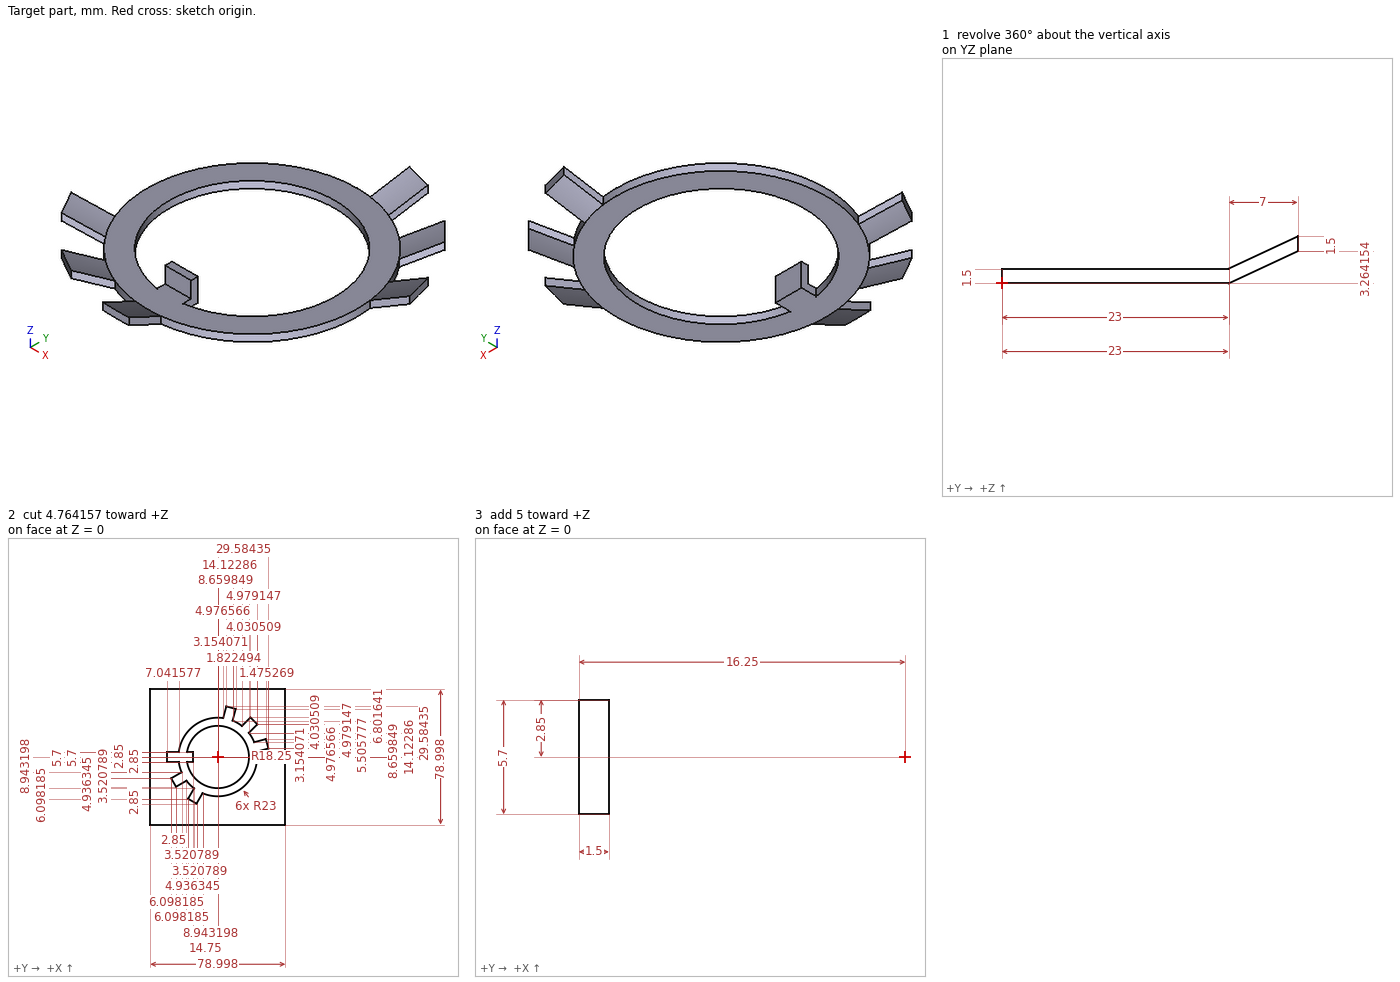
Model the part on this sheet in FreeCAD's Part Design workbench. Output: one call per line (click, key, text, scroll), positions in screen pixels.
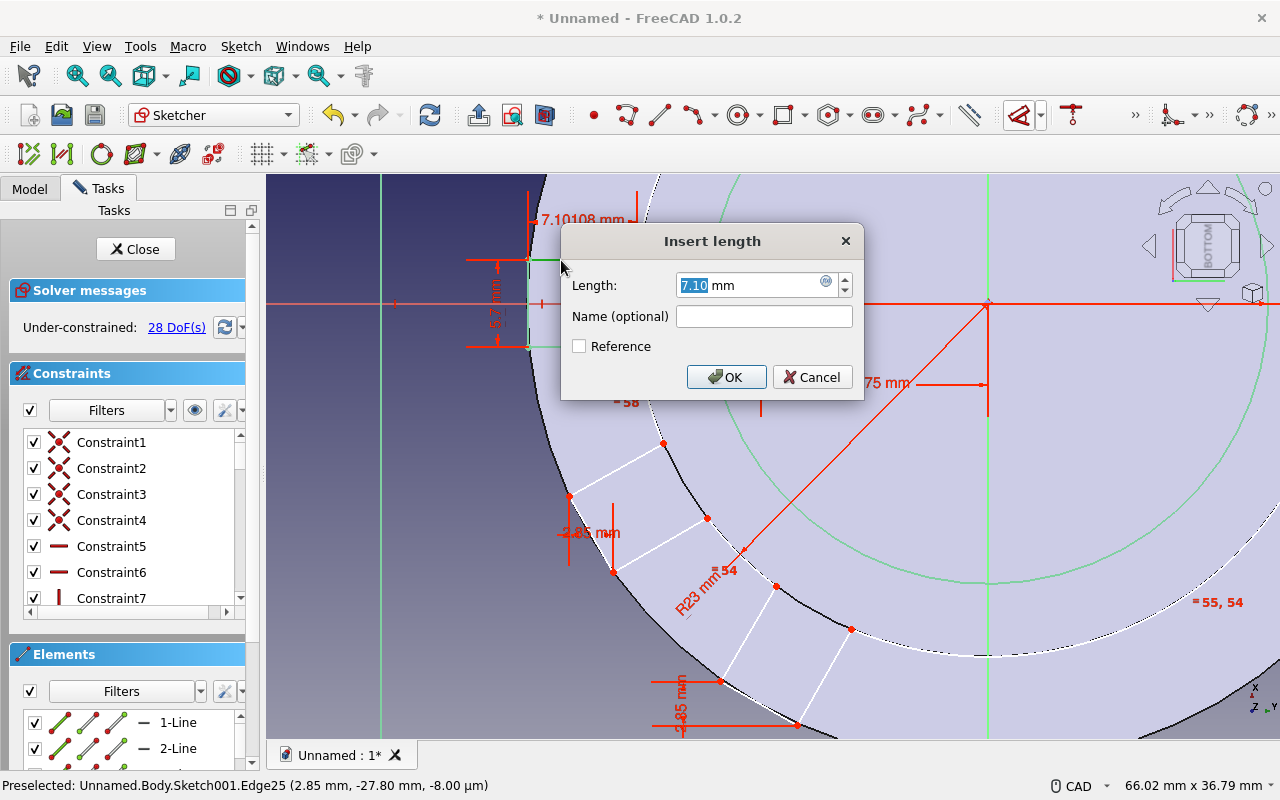
text(7.041577)
key(Return)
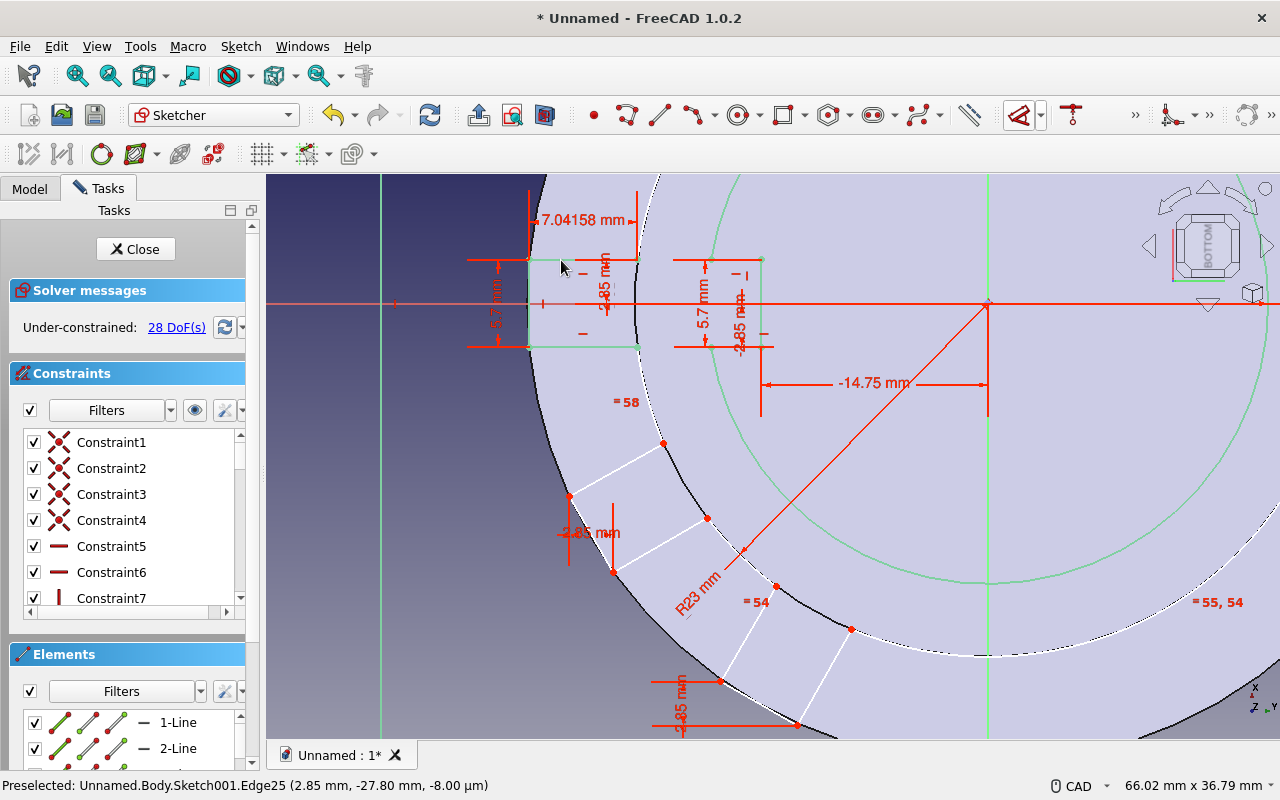
click(664, 444)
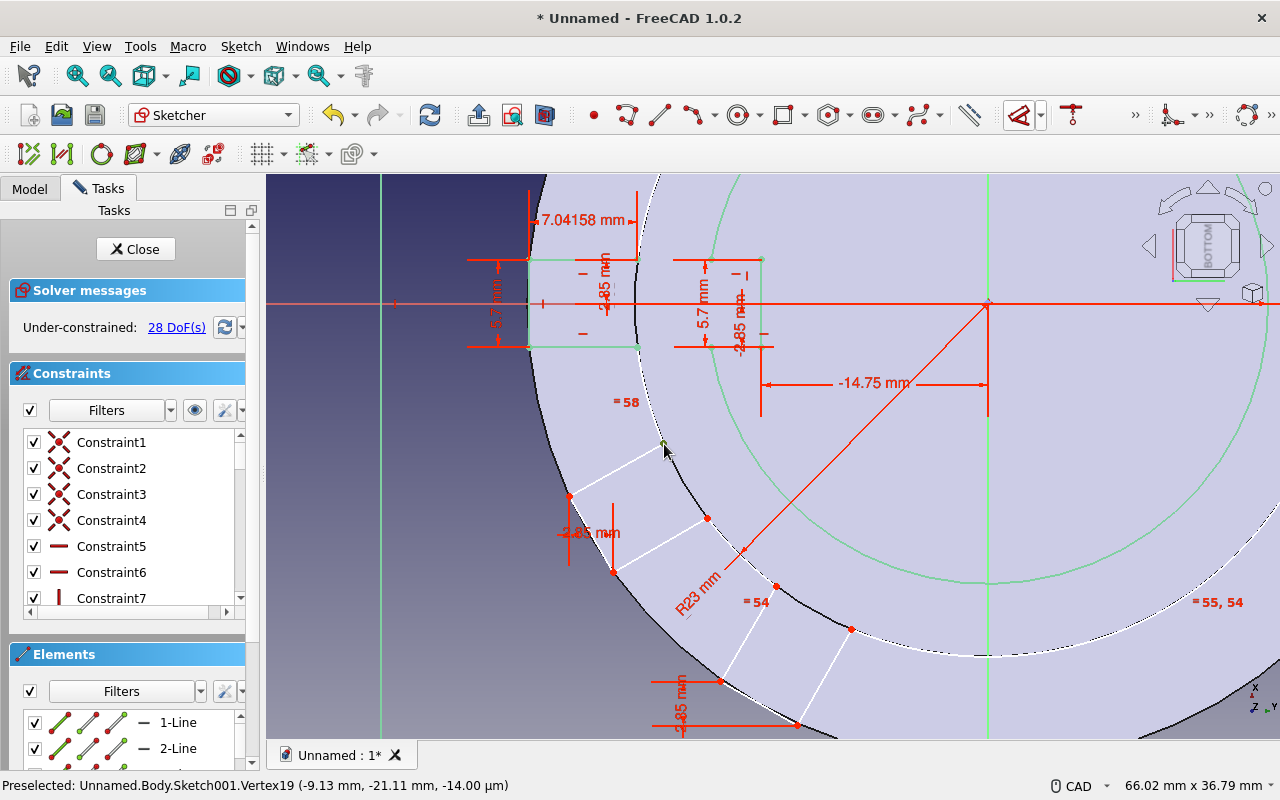
click(1040, 116)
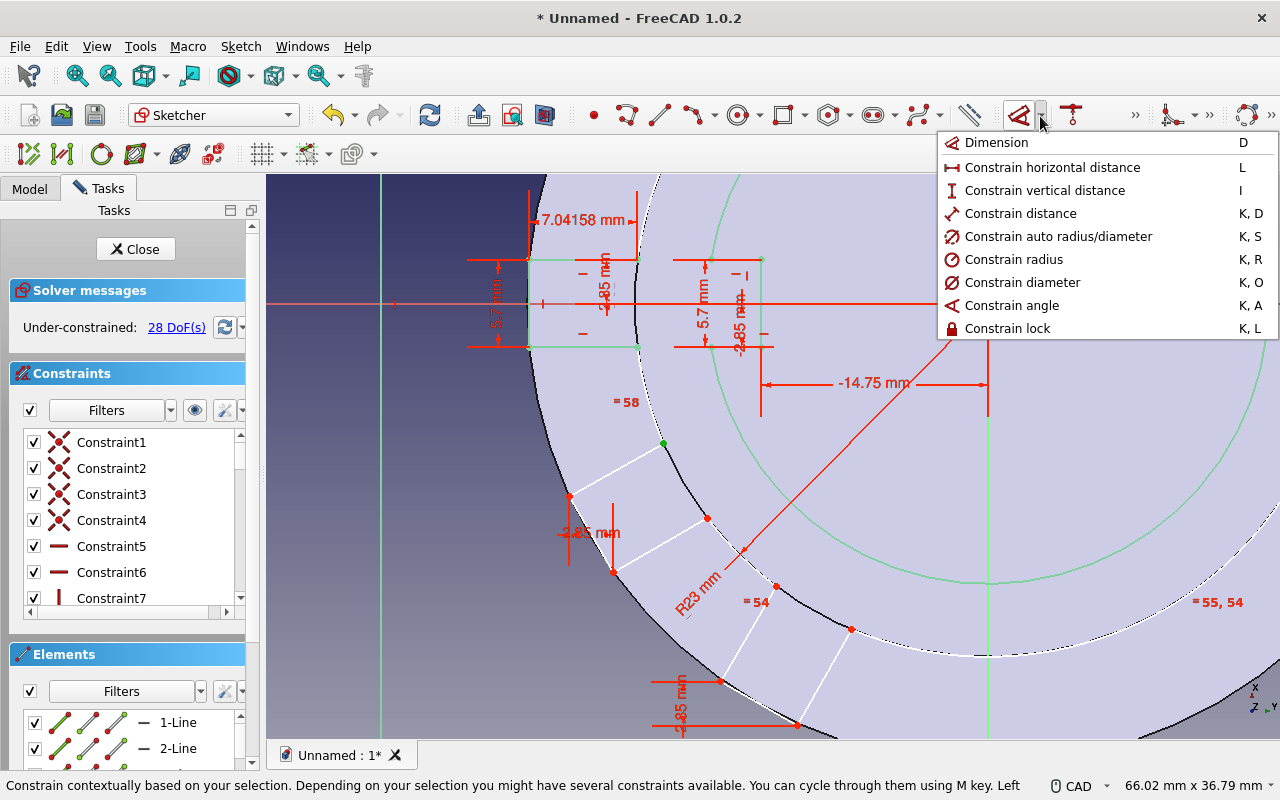
click(1108, 190)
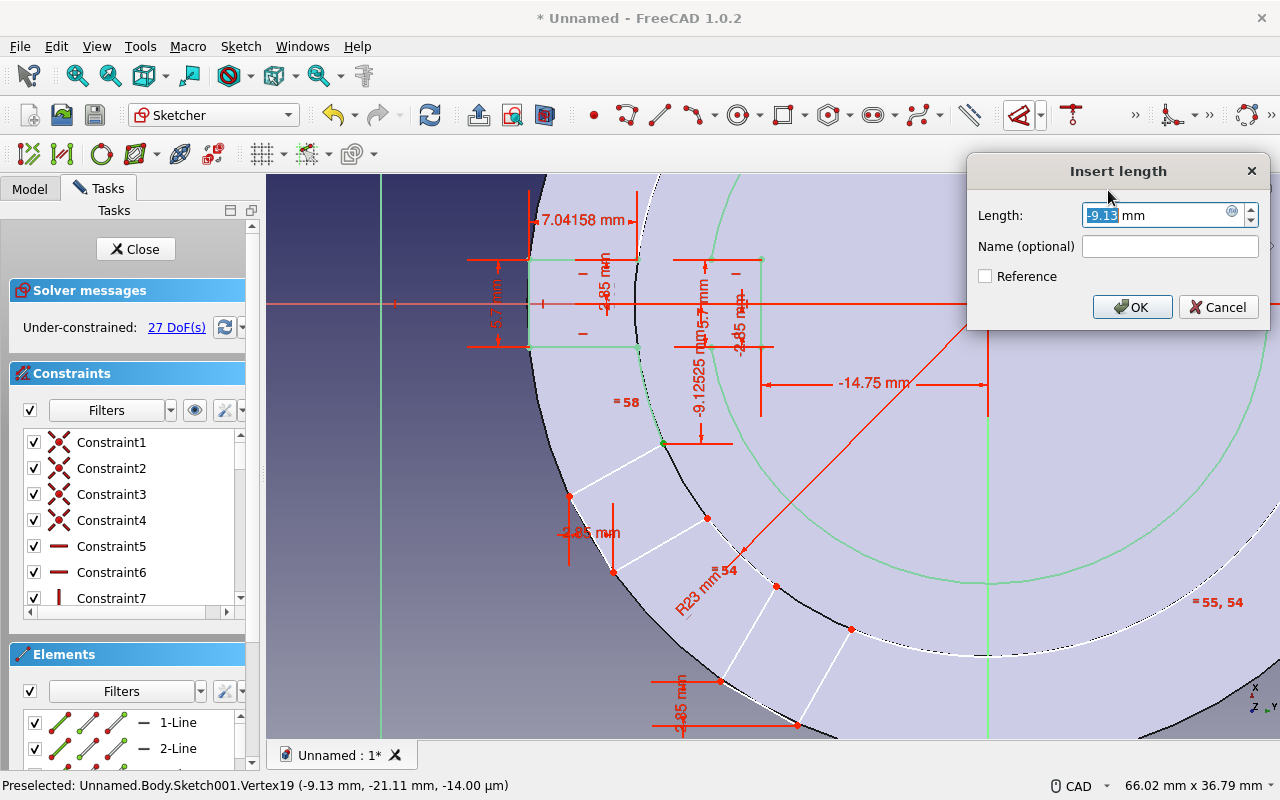
text(-8.943198)
key(Return)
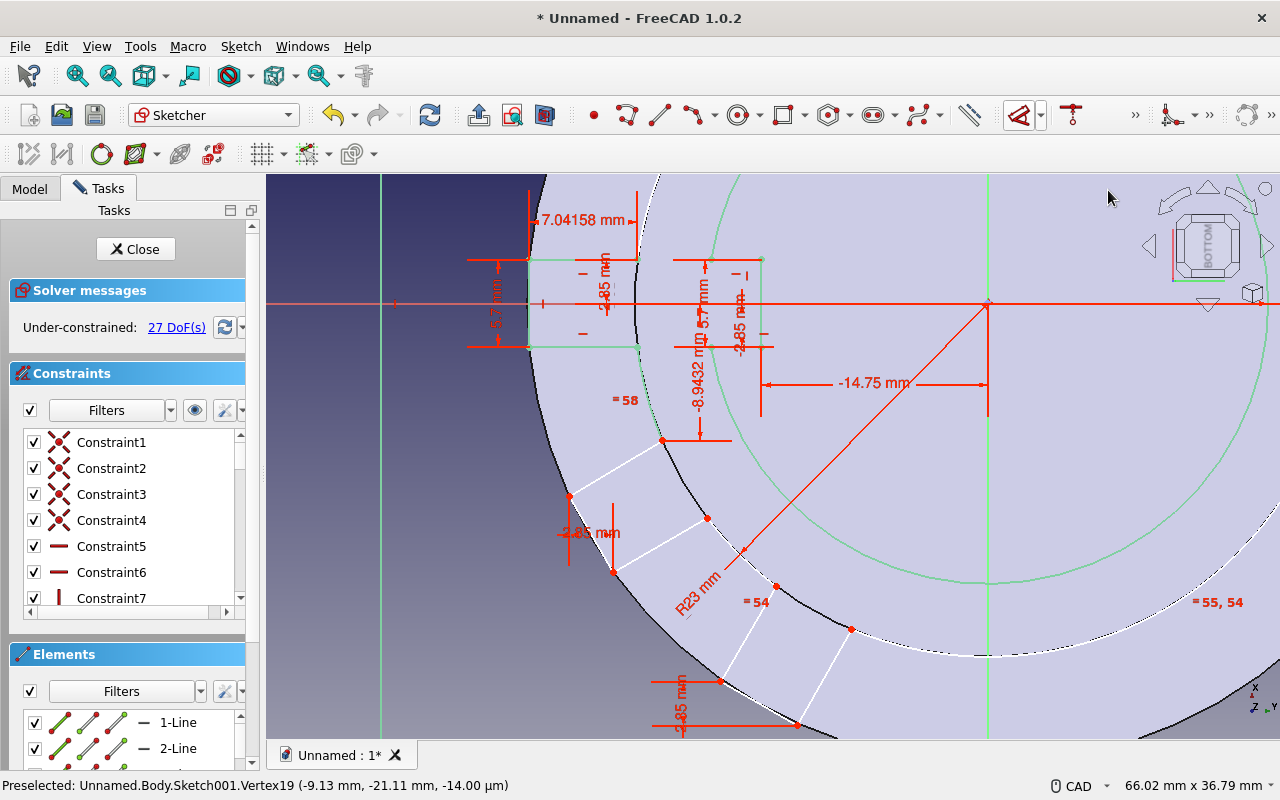
click(852, 630)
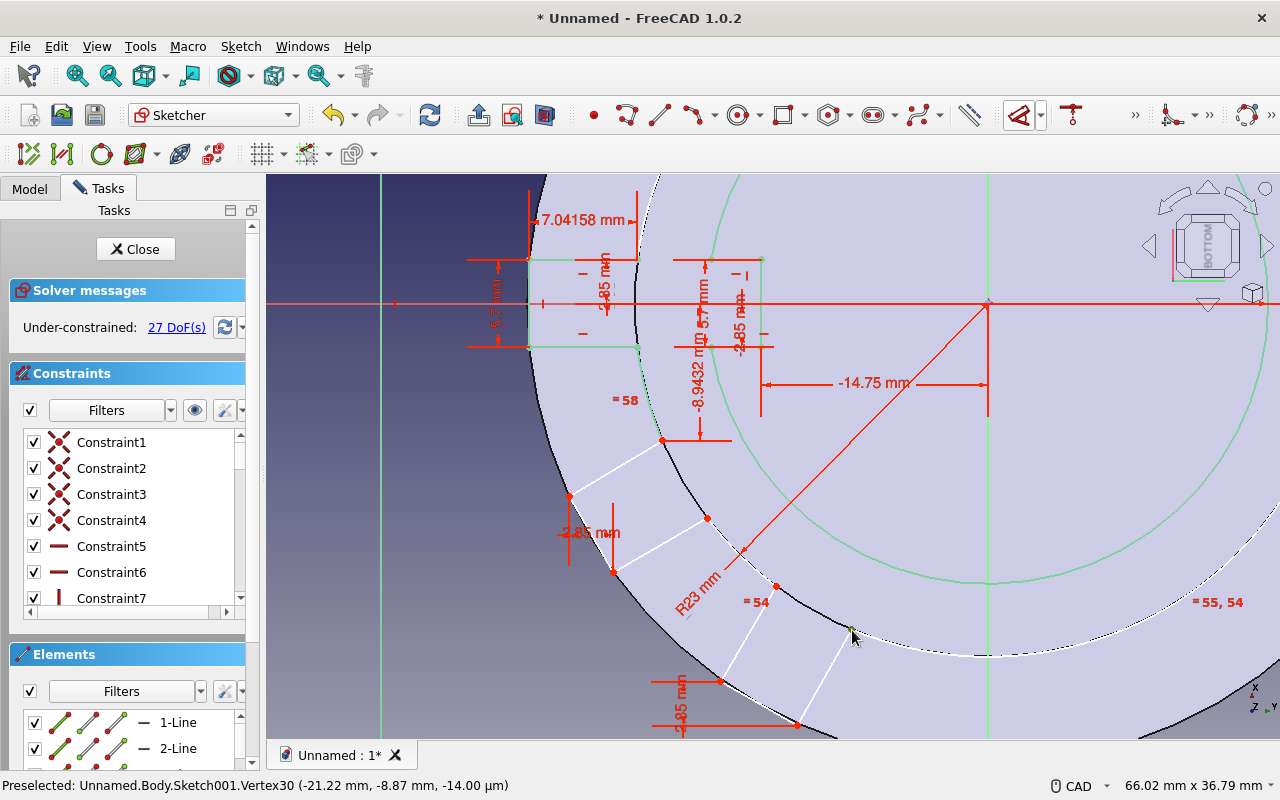
click(1040, 116)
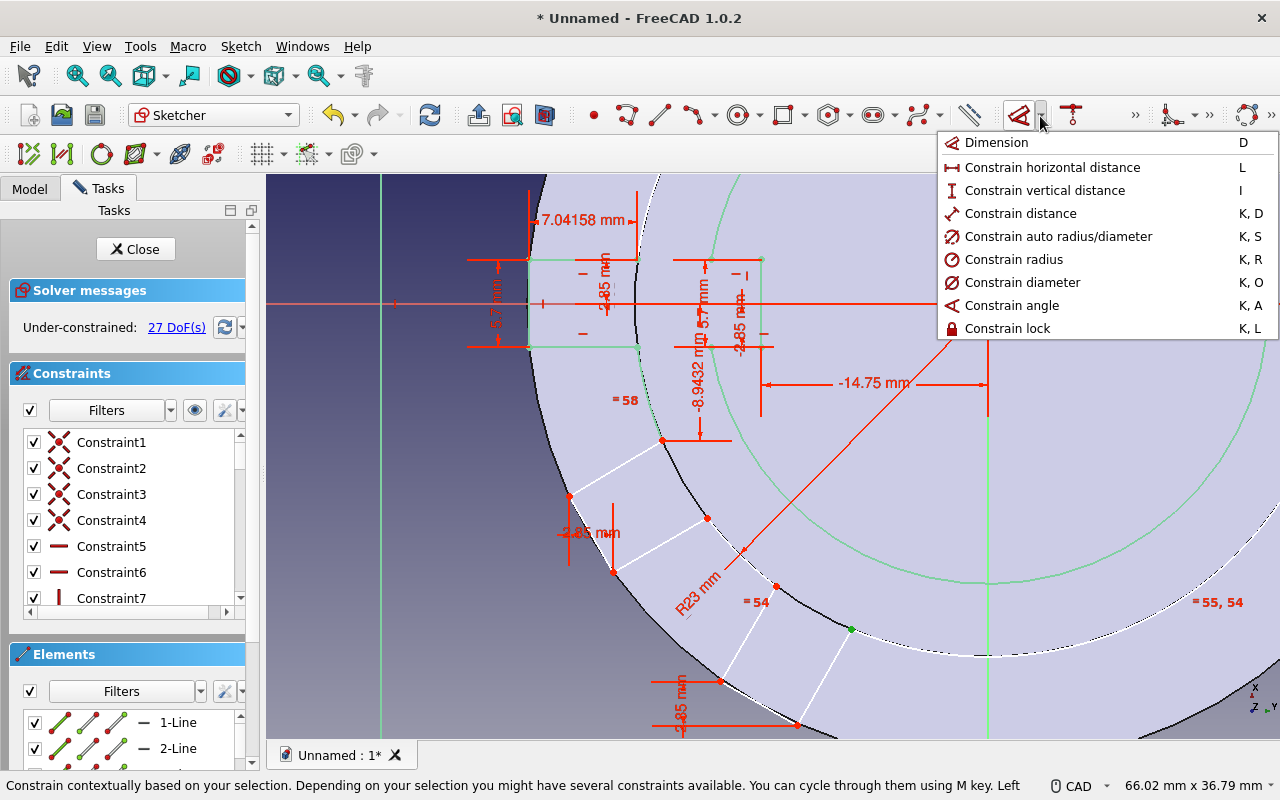
click(1108, 168)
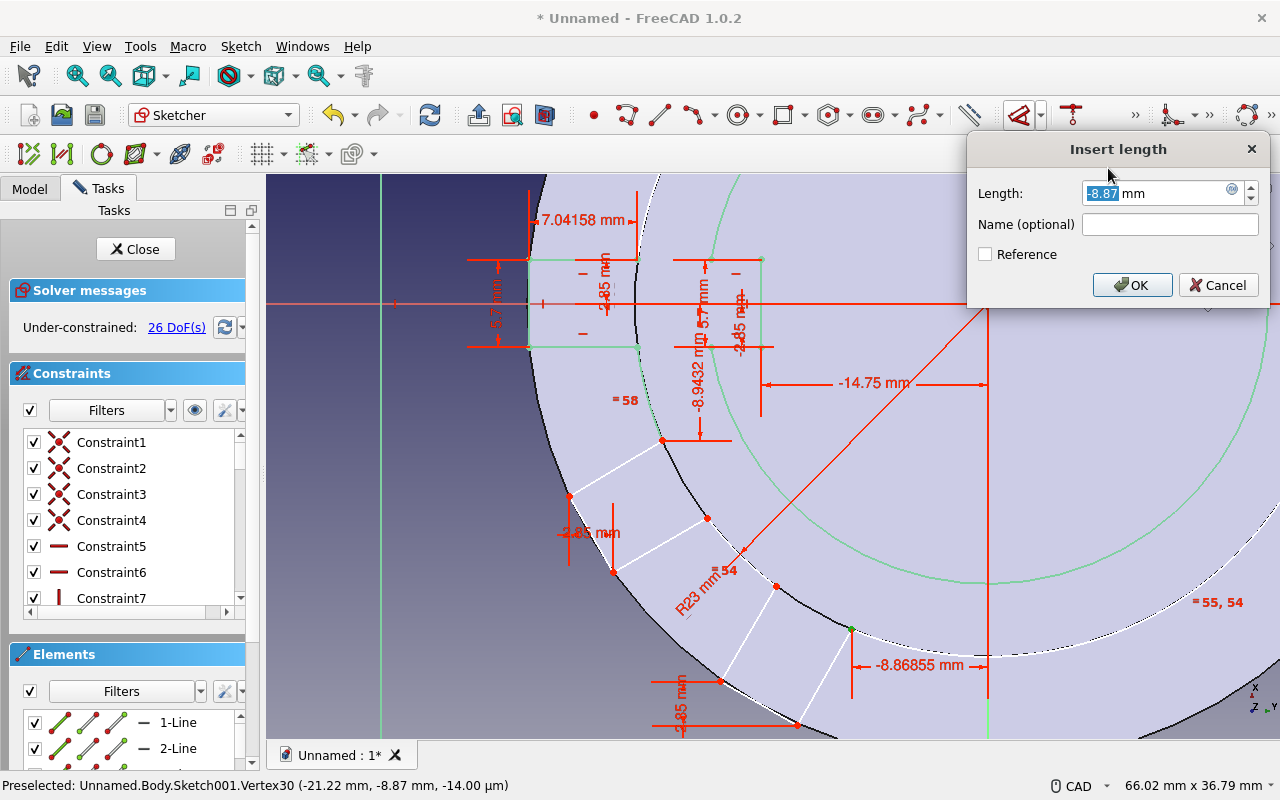
text(-8.943198)
key(Return)